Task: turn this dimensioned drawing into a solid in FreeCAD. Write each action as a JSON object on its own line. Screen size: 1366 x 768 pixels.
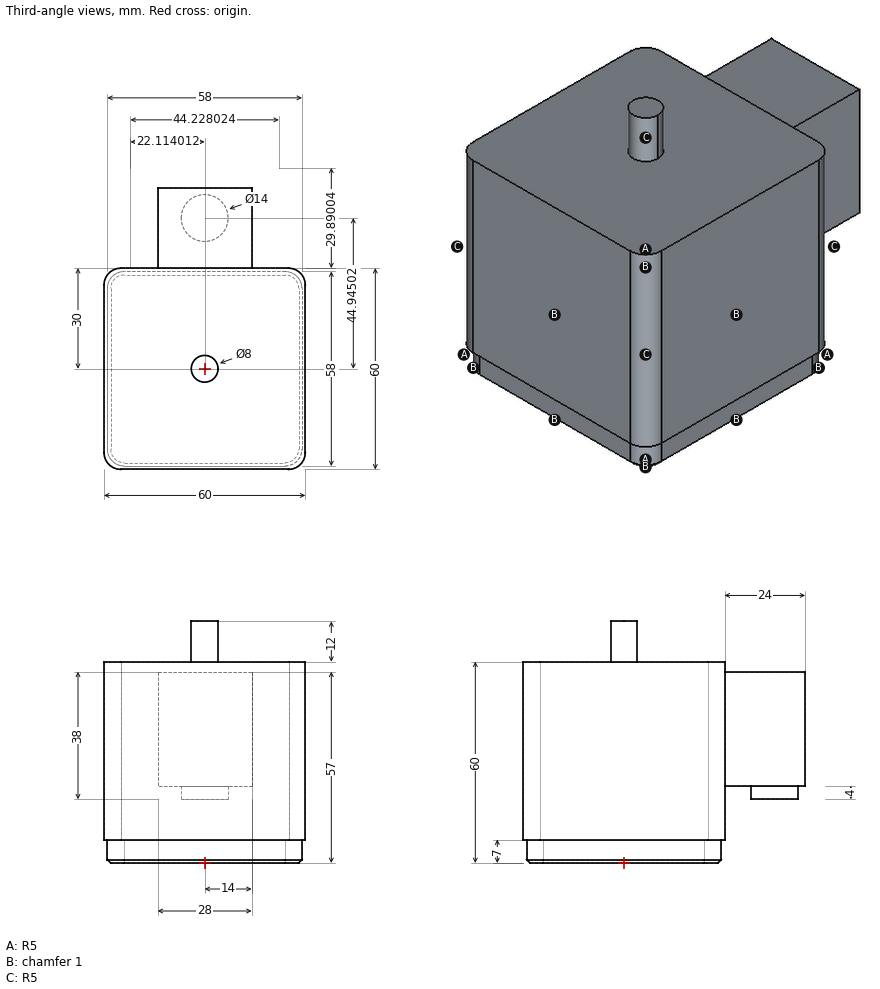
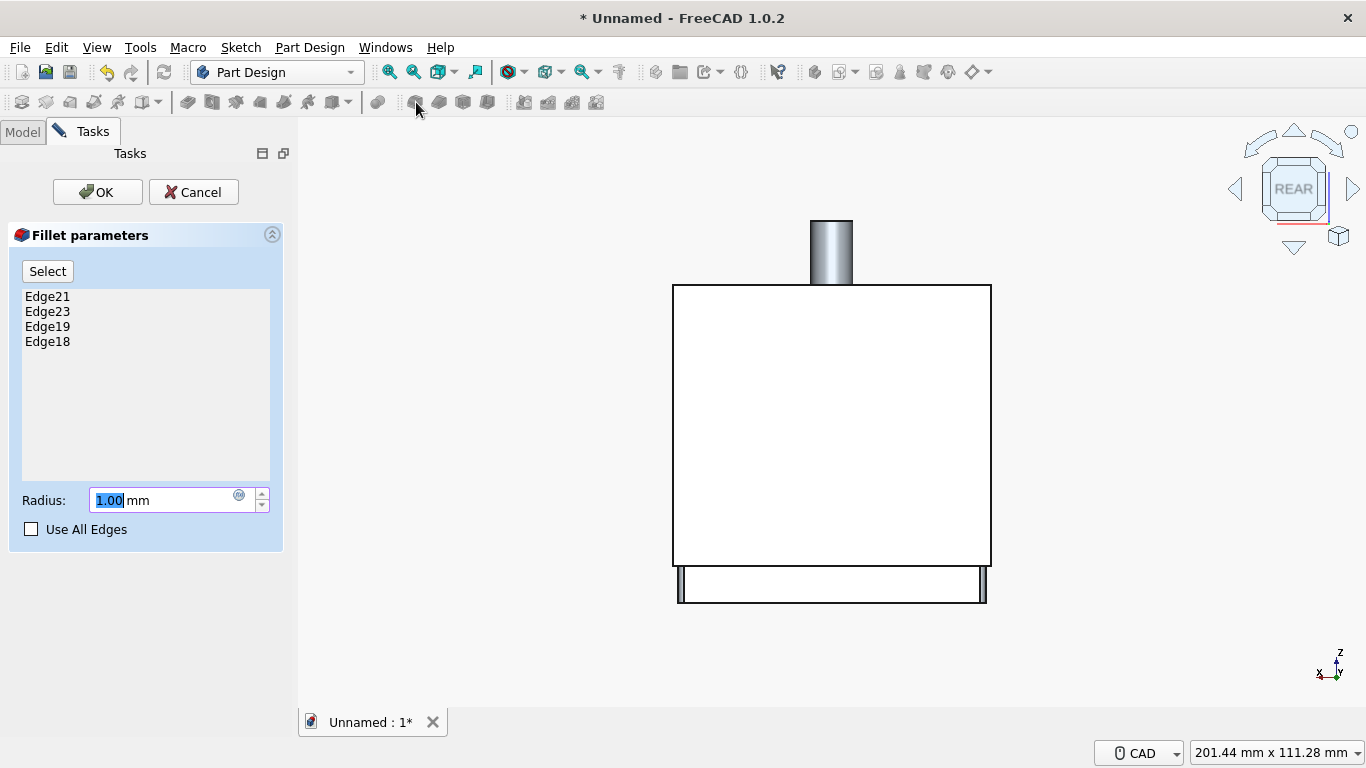
{"action": "type", "text": "5"}
{"action": "key", "text": "Tab"}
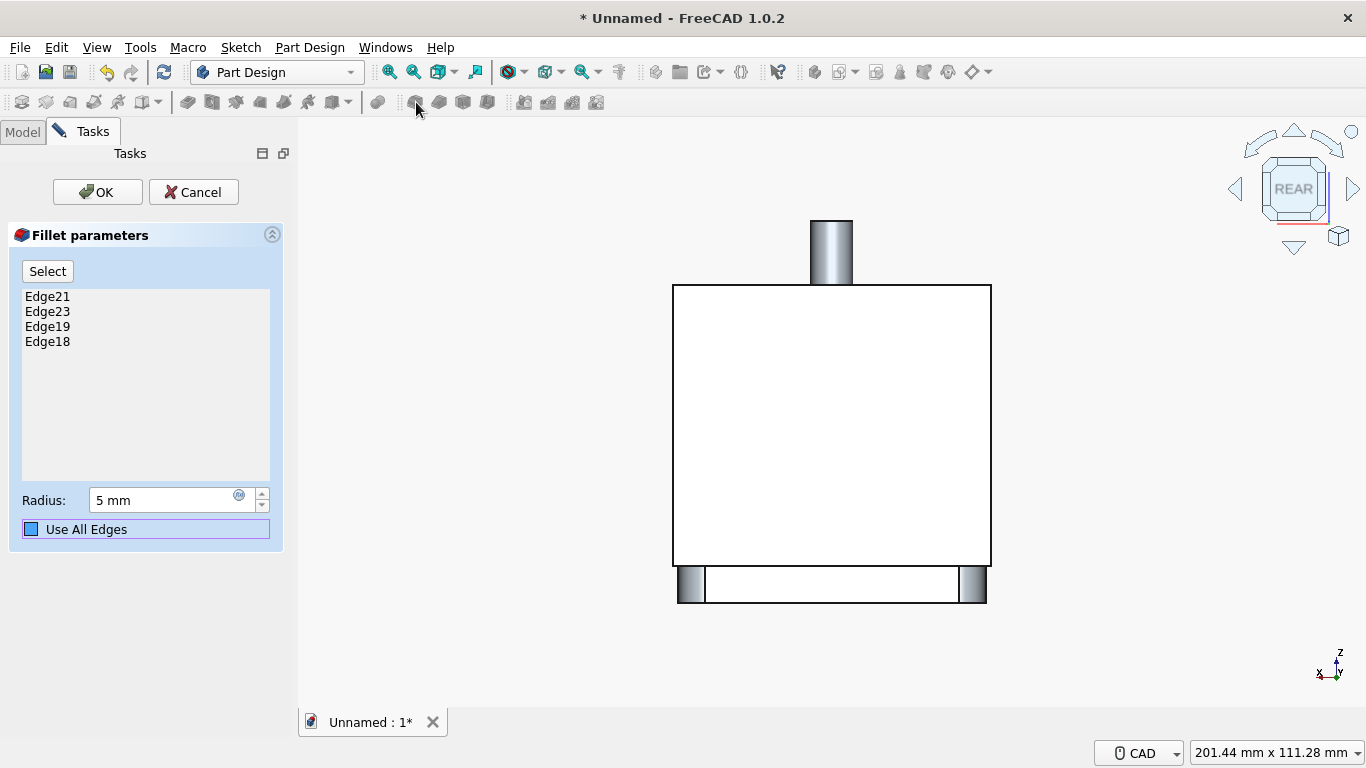
{"action": "left_click", "coordinate": [98, 192]}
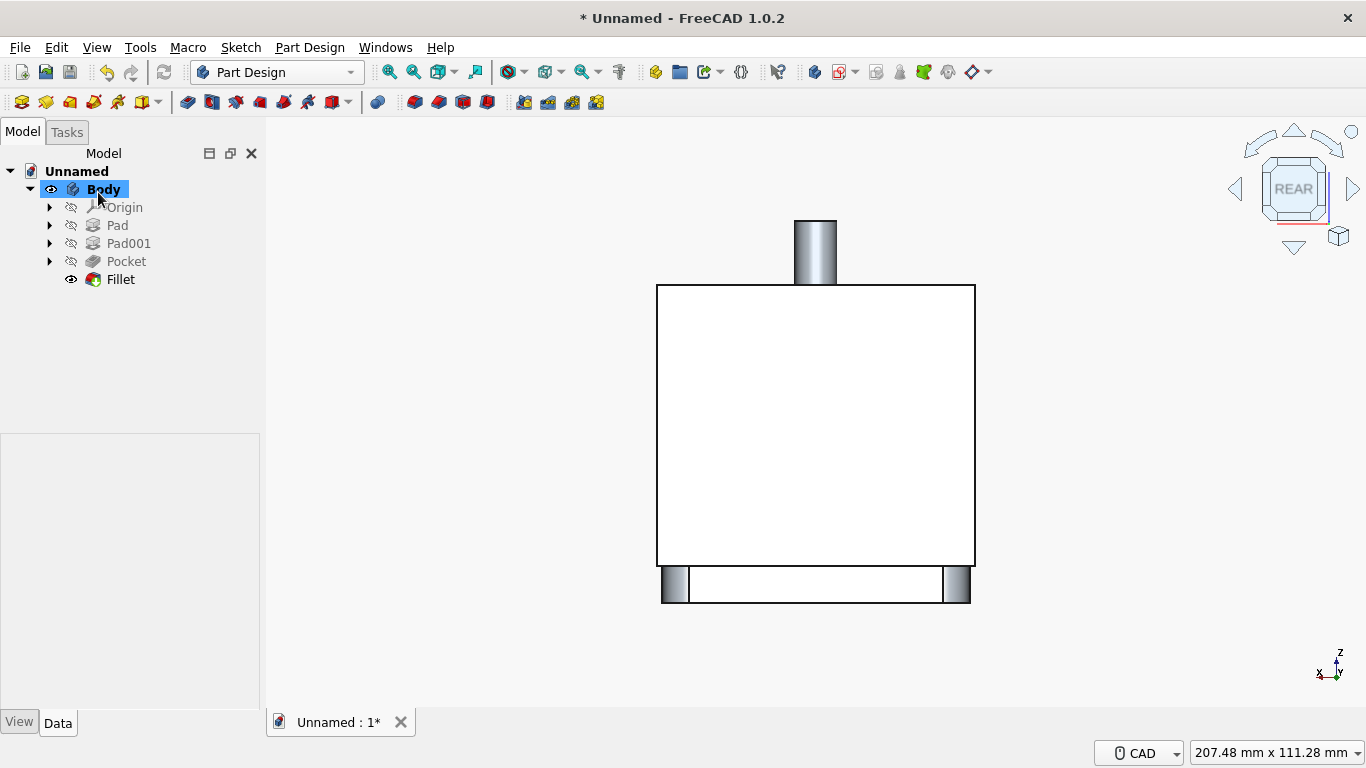
{"action": "key", "text": "0"}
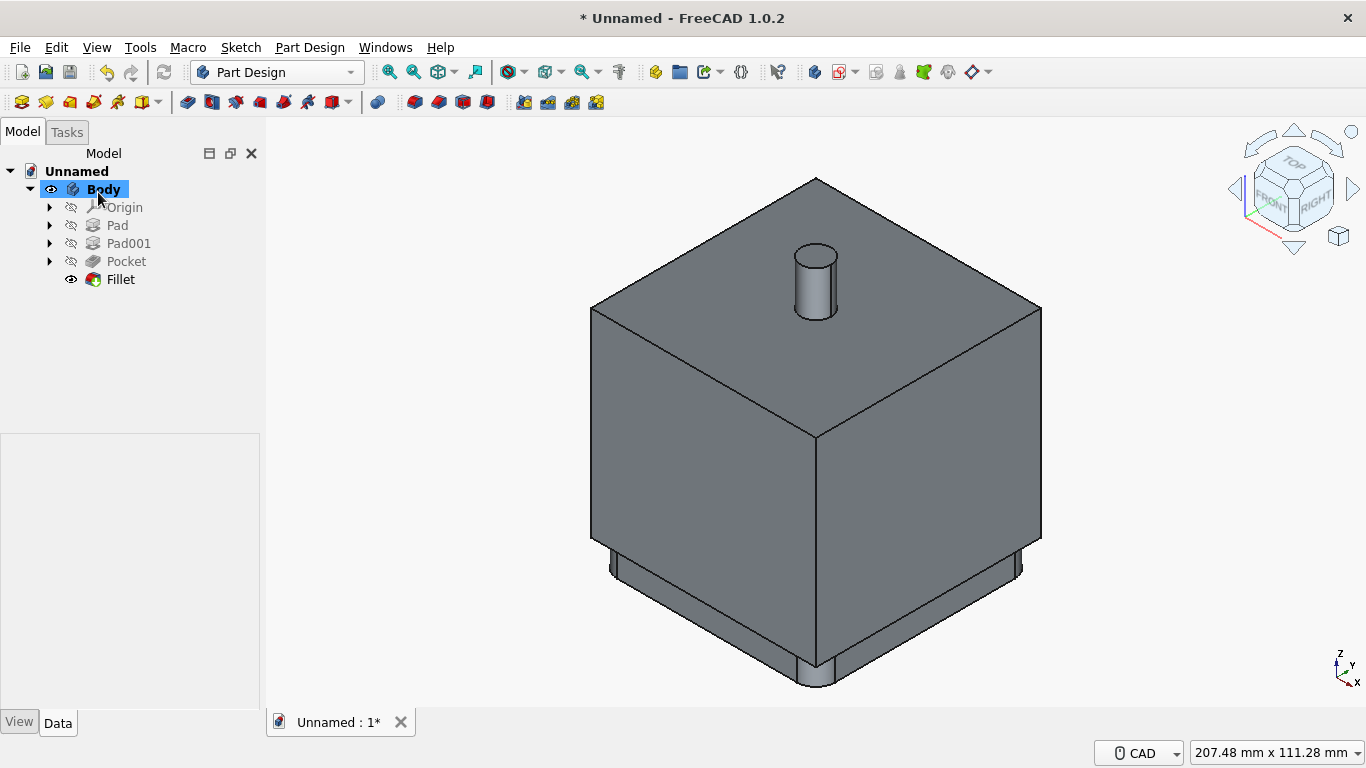
{"action": "key", "text": "2"}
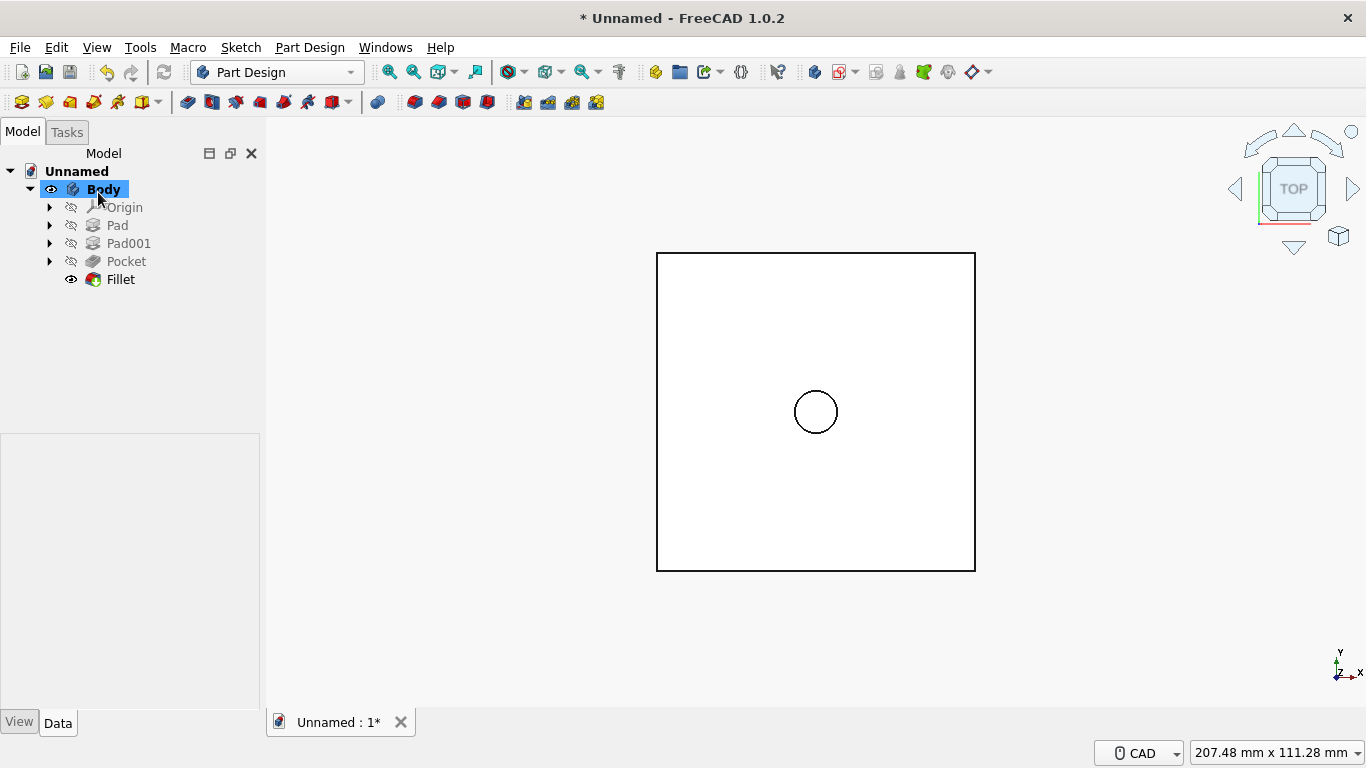
{"action": "key", "text": "1"}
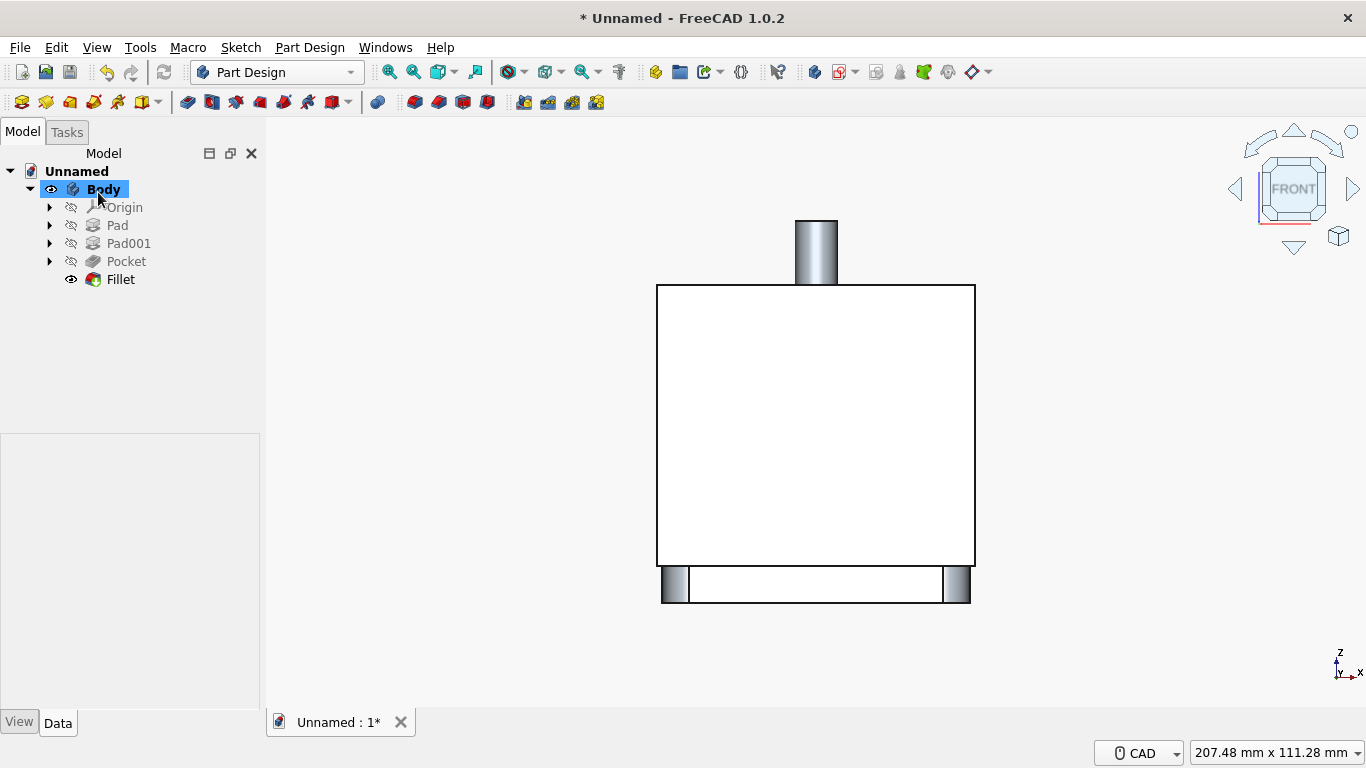
{"action": "key", "text": "3"}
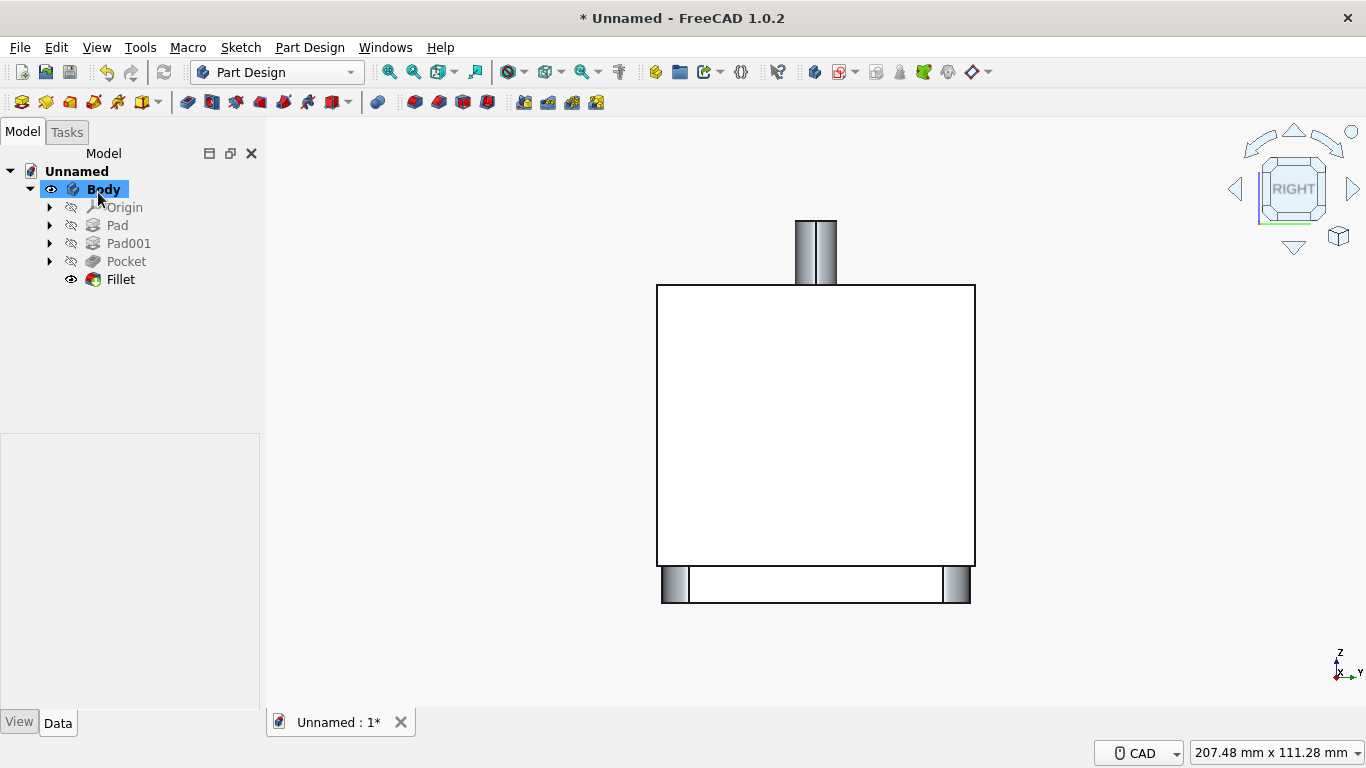
{"action": "key", "text": "5"}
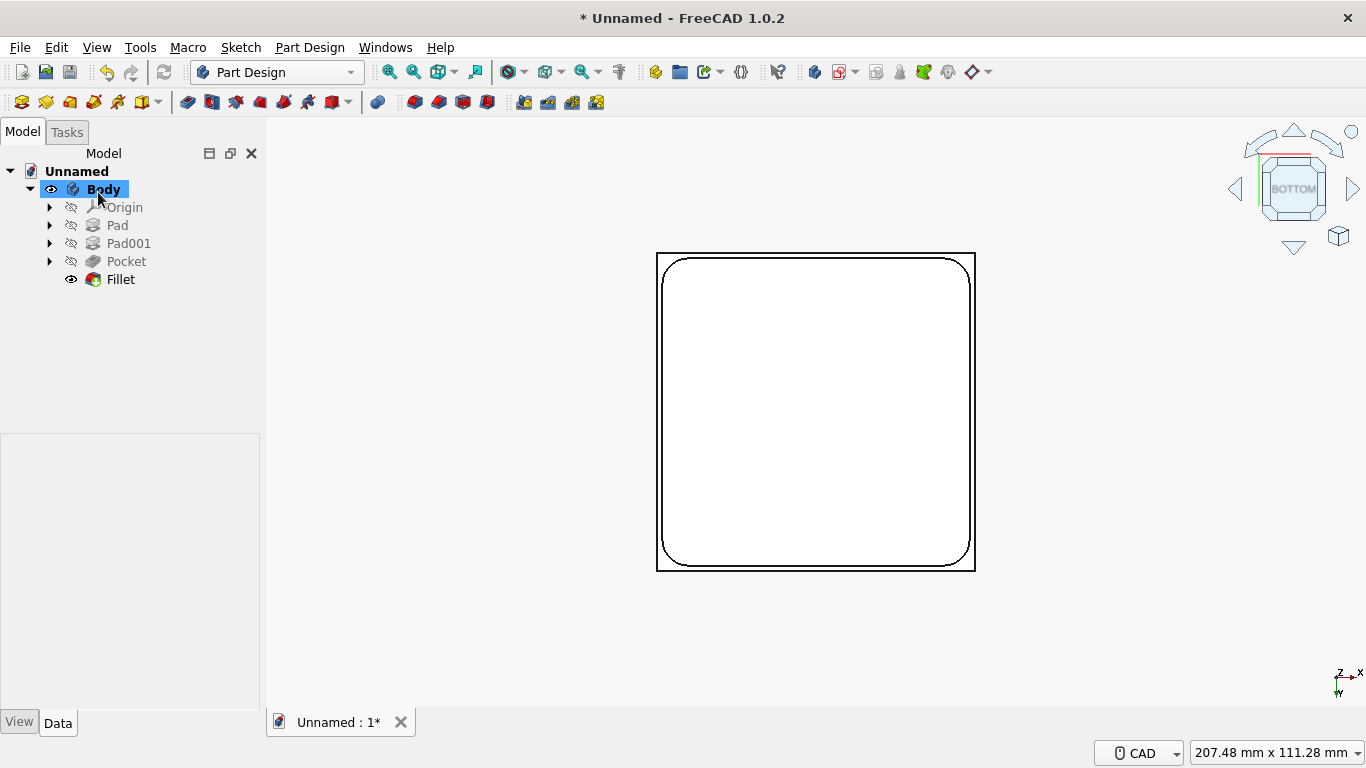
{"action": "left_click", "coordinate": [816, 411]}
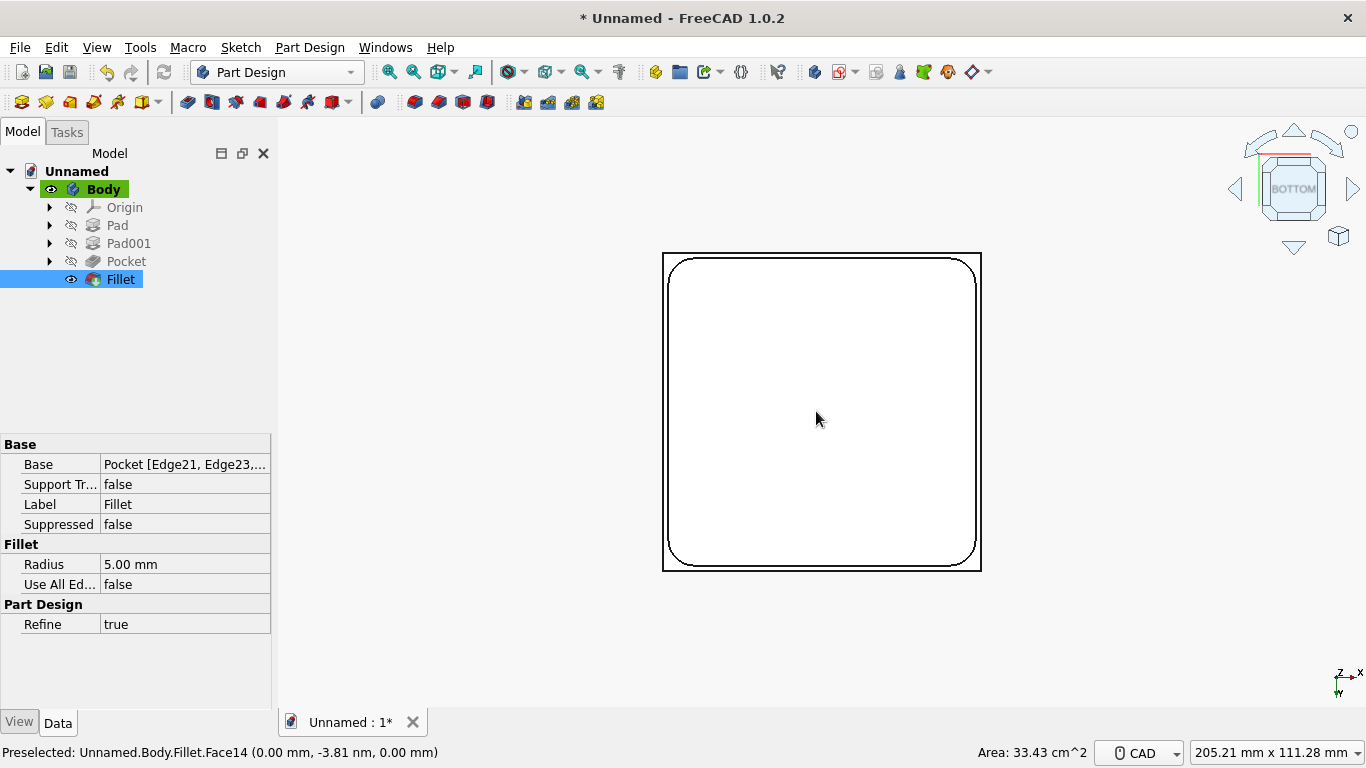
{"action": "left_click", "coordinate": [440, 102]}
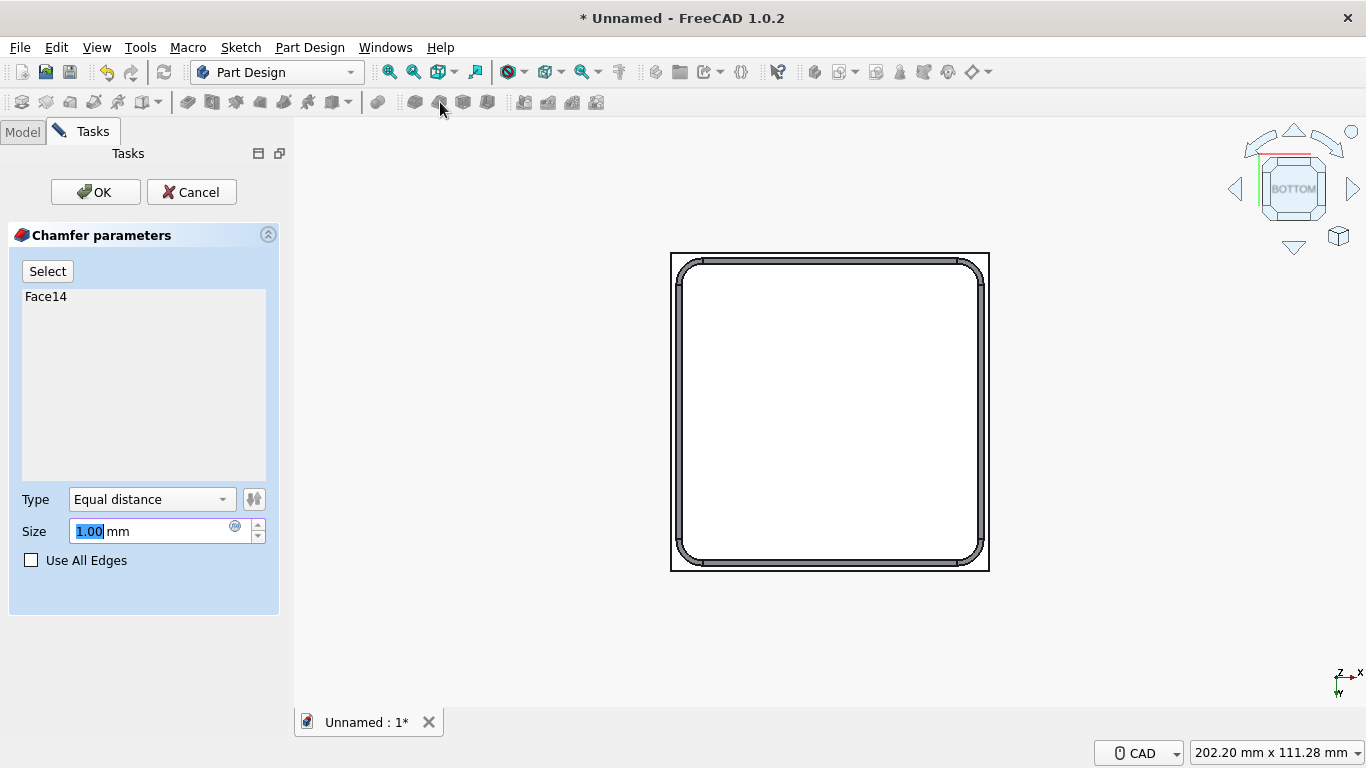
{"action": "type", "text": "1"}
{"action": "key", "text": "Tab"}